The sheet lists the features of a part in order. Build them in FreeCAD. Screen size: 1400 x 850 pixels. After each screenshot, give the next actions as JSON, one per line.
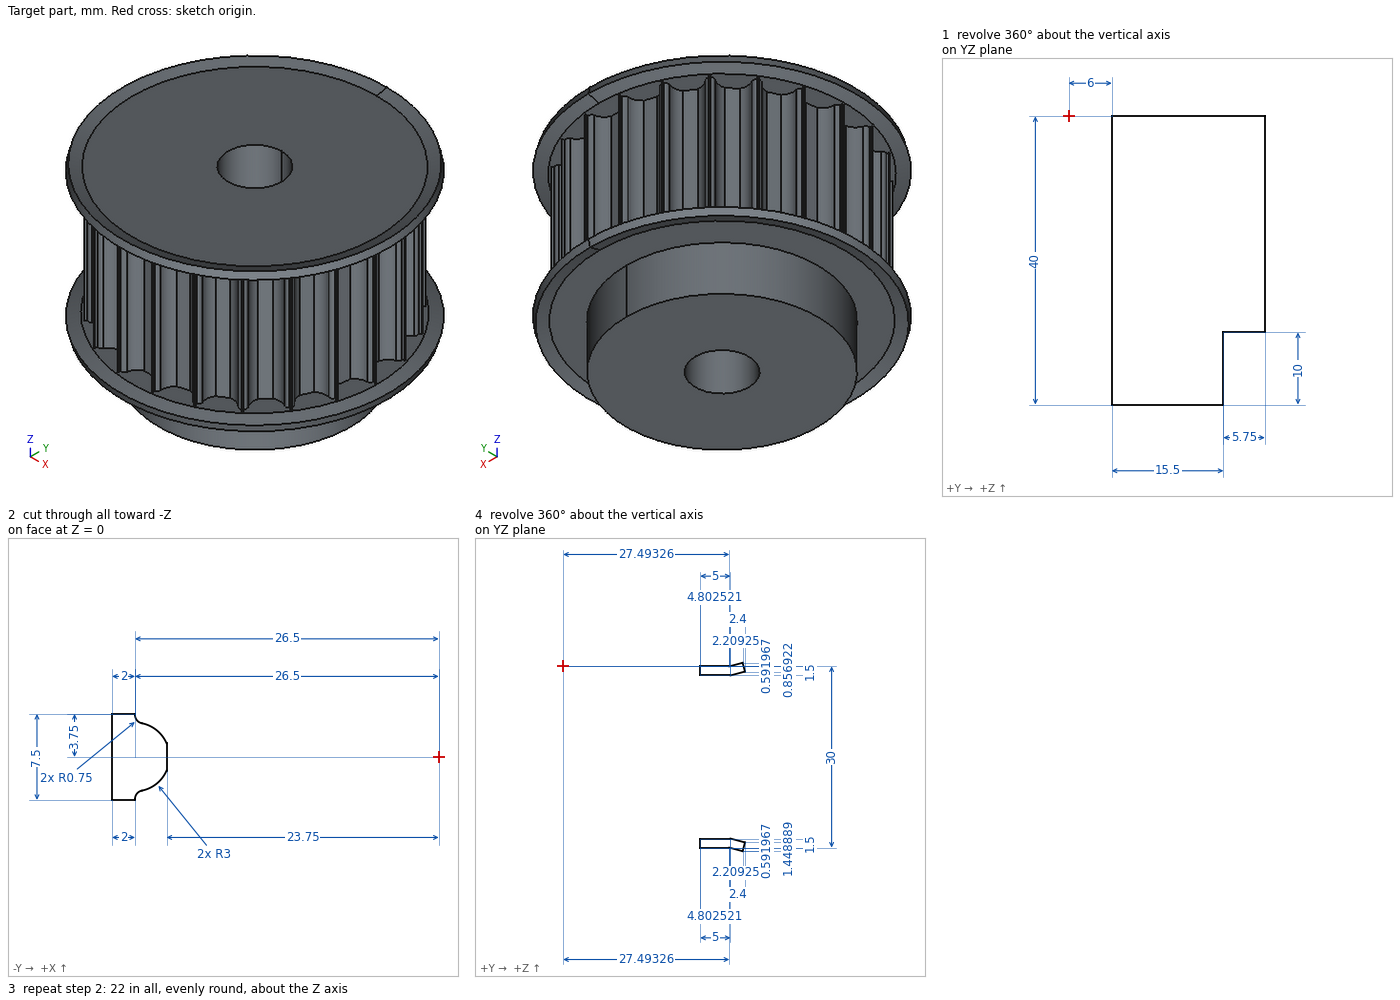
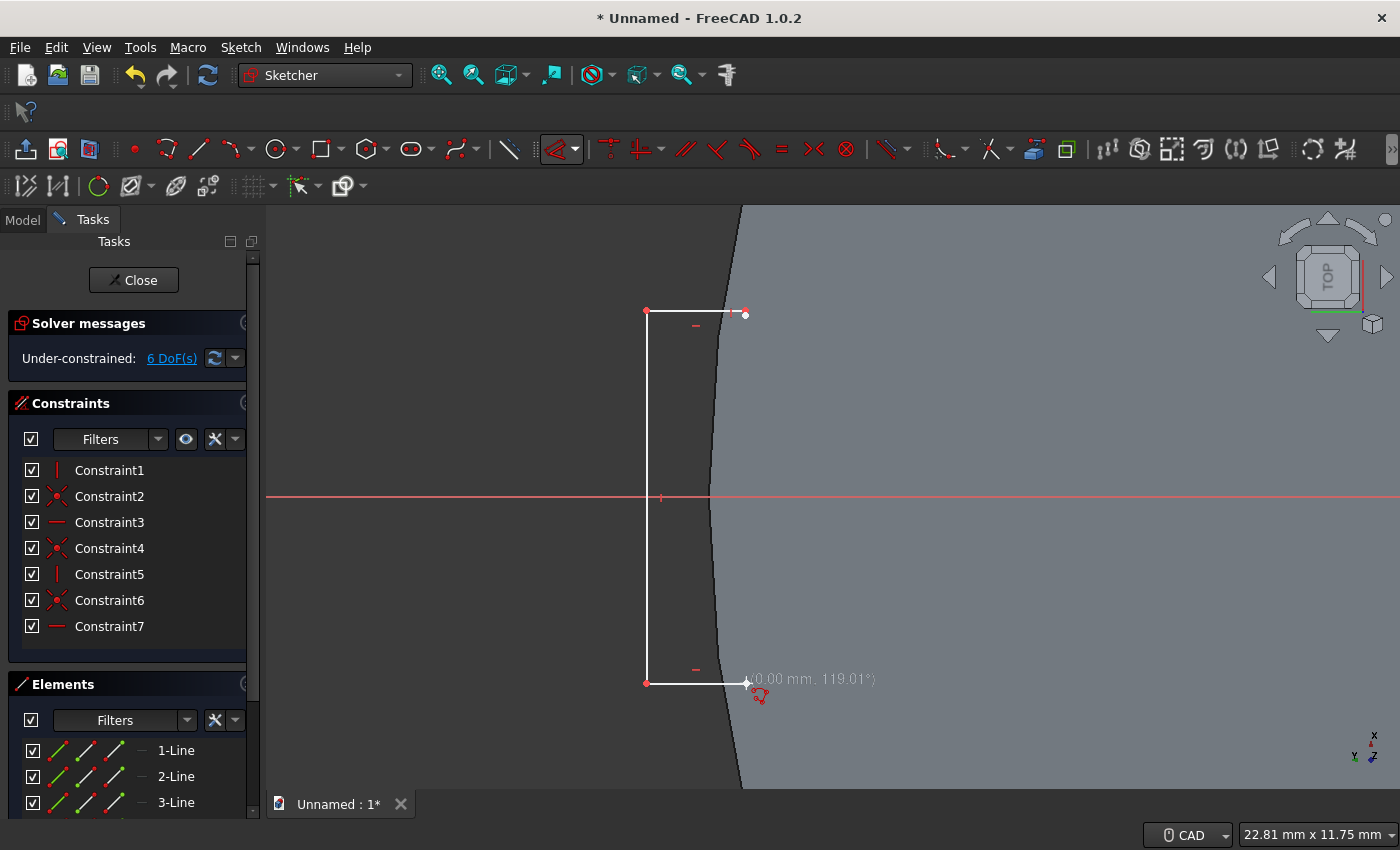
{"action": "scroll", "coordinate": [746, 680], "scroll_direction": "up", "scroll_amount": 8}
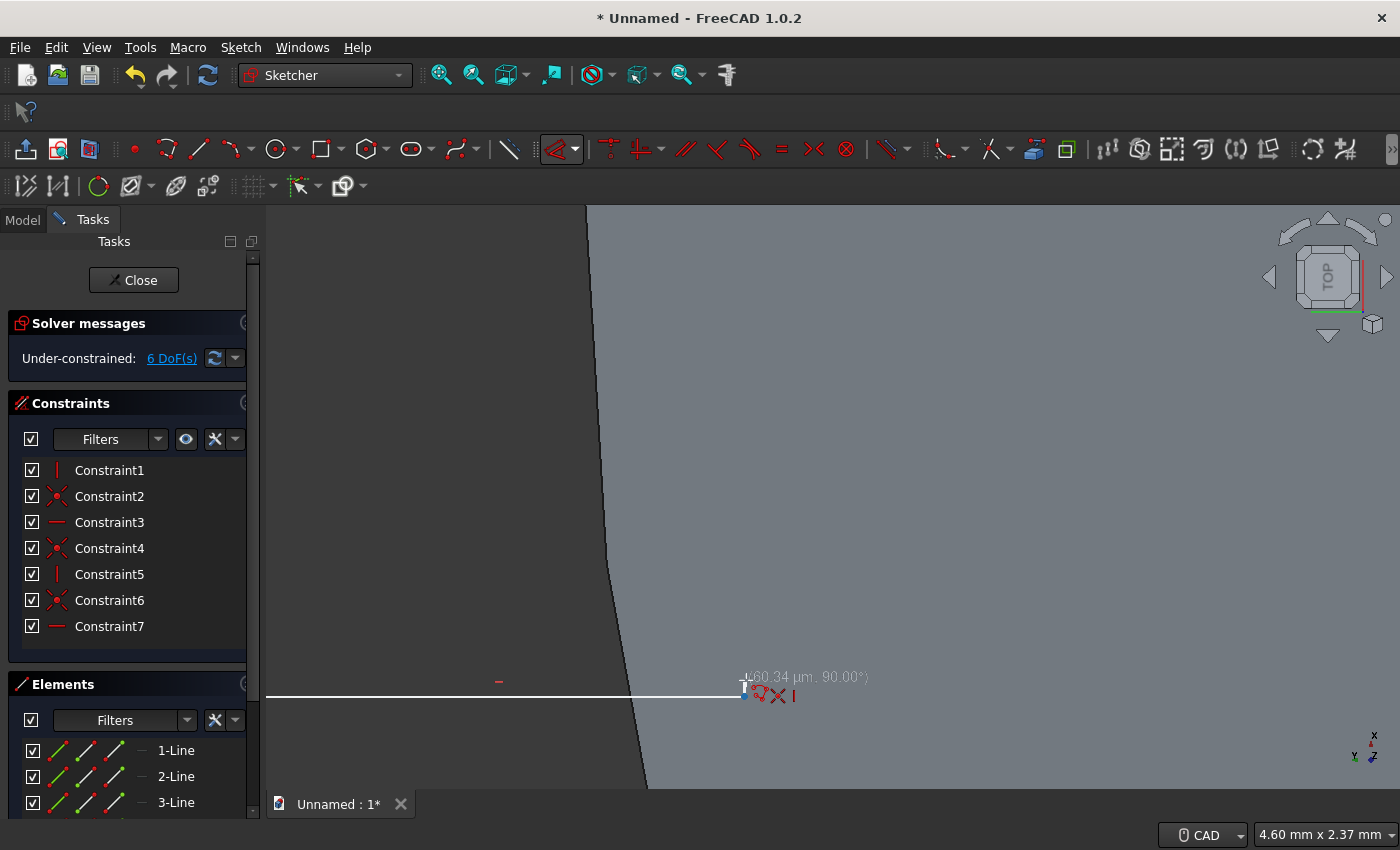
{"action": "left_click", "coordinate": [744, 675]}
{"action": "right_click", "coordinate": [744, 675]}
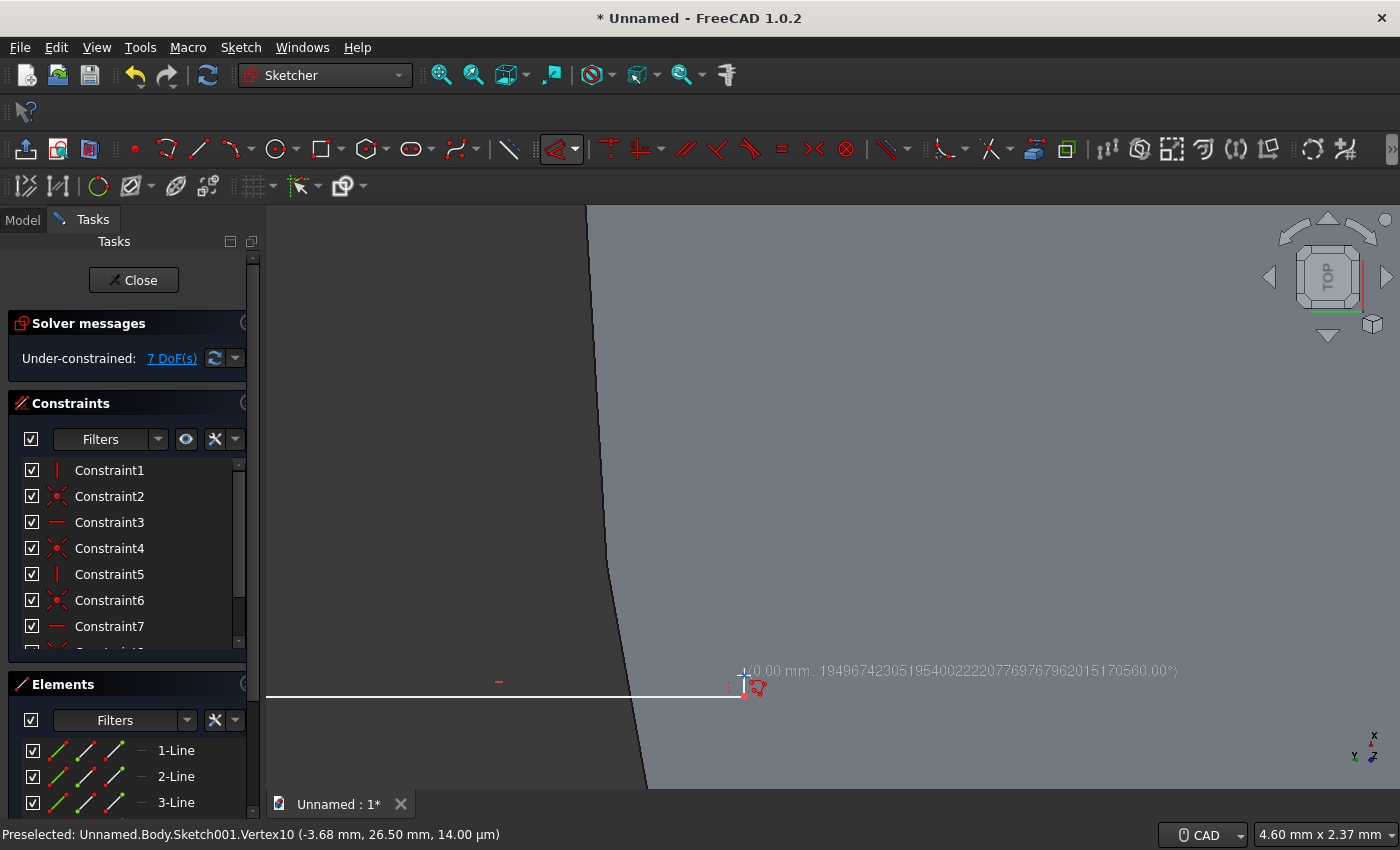
{"action": "key", "text": "g l"}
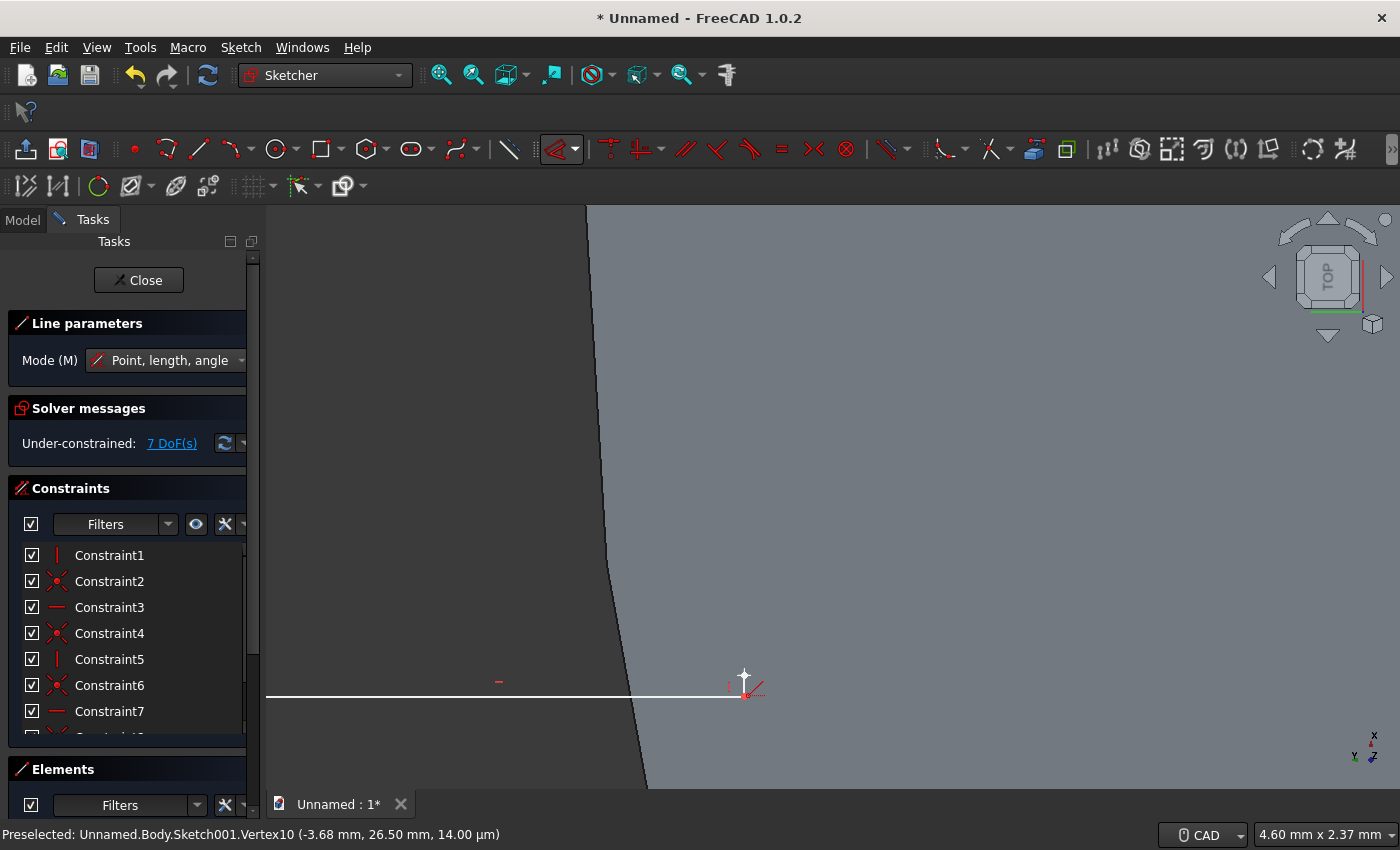
{"action": "scroll", "coordinate": [746, 681], "scroll_direction": "down", "scroll_amount": 8}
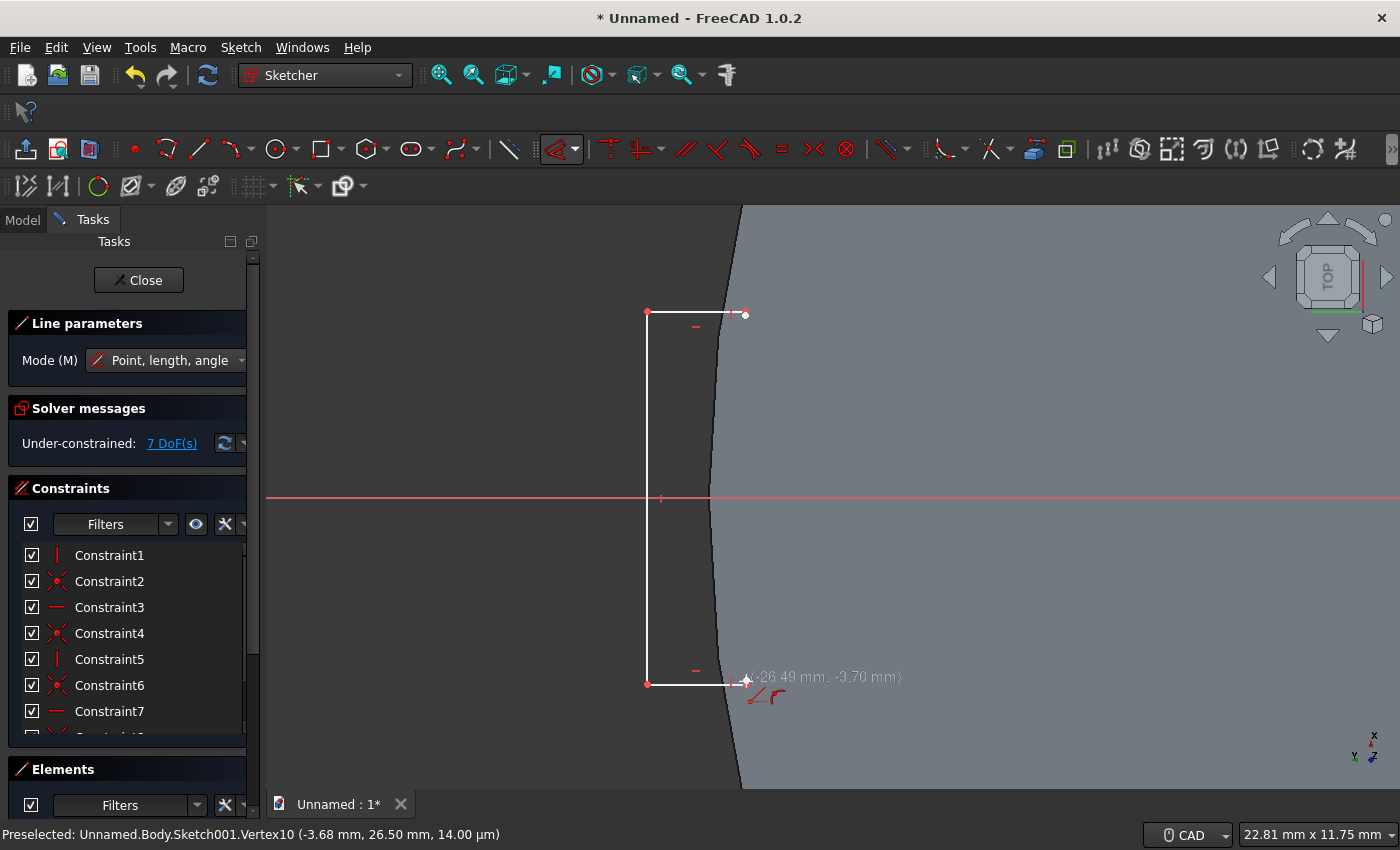
{"action": "left_click", "coordinate": [883, 557]}
{"action": "left_click", "coordinate": [883, 438]}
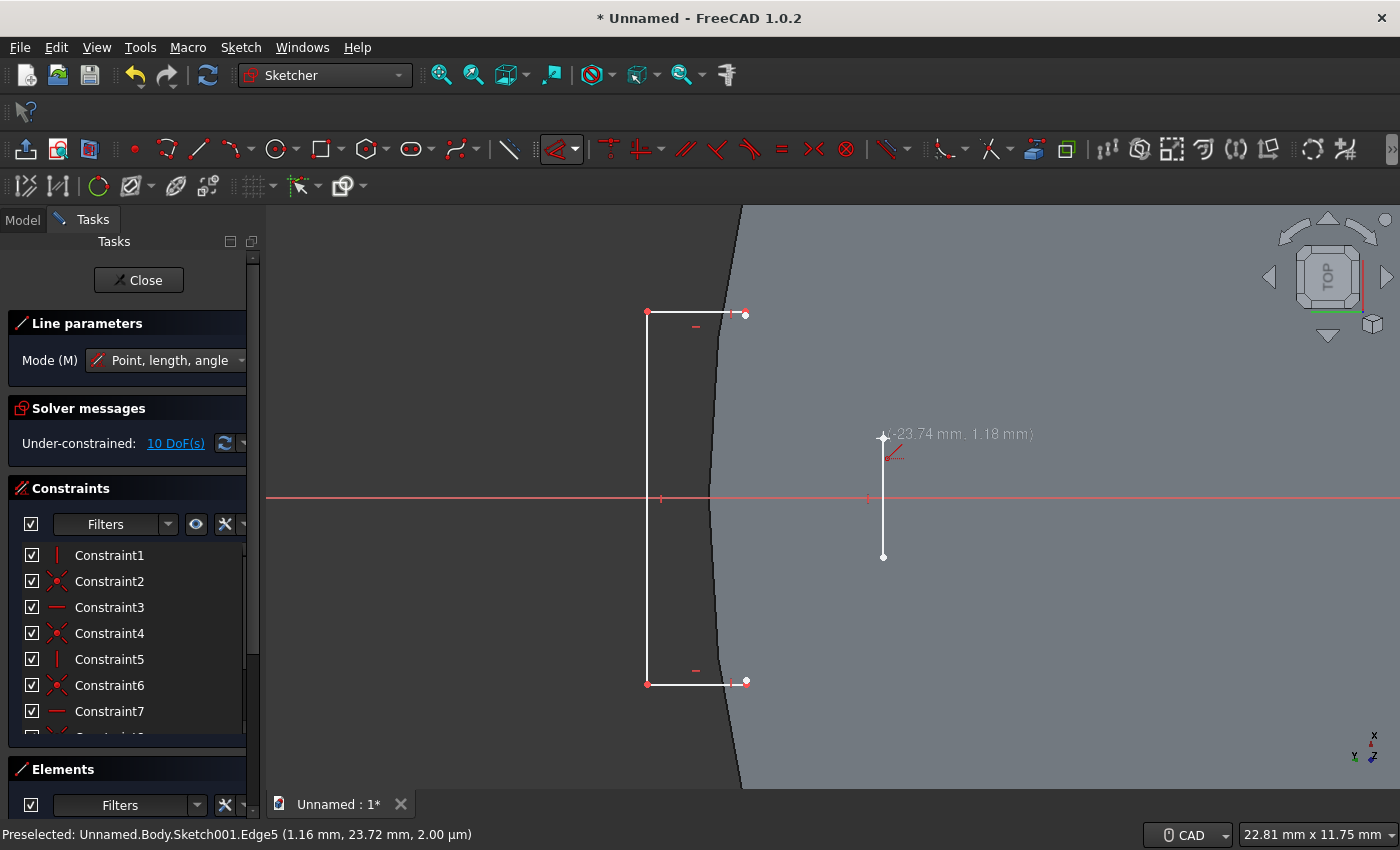
{"action": "left_click", "coordinate": [232, 150]}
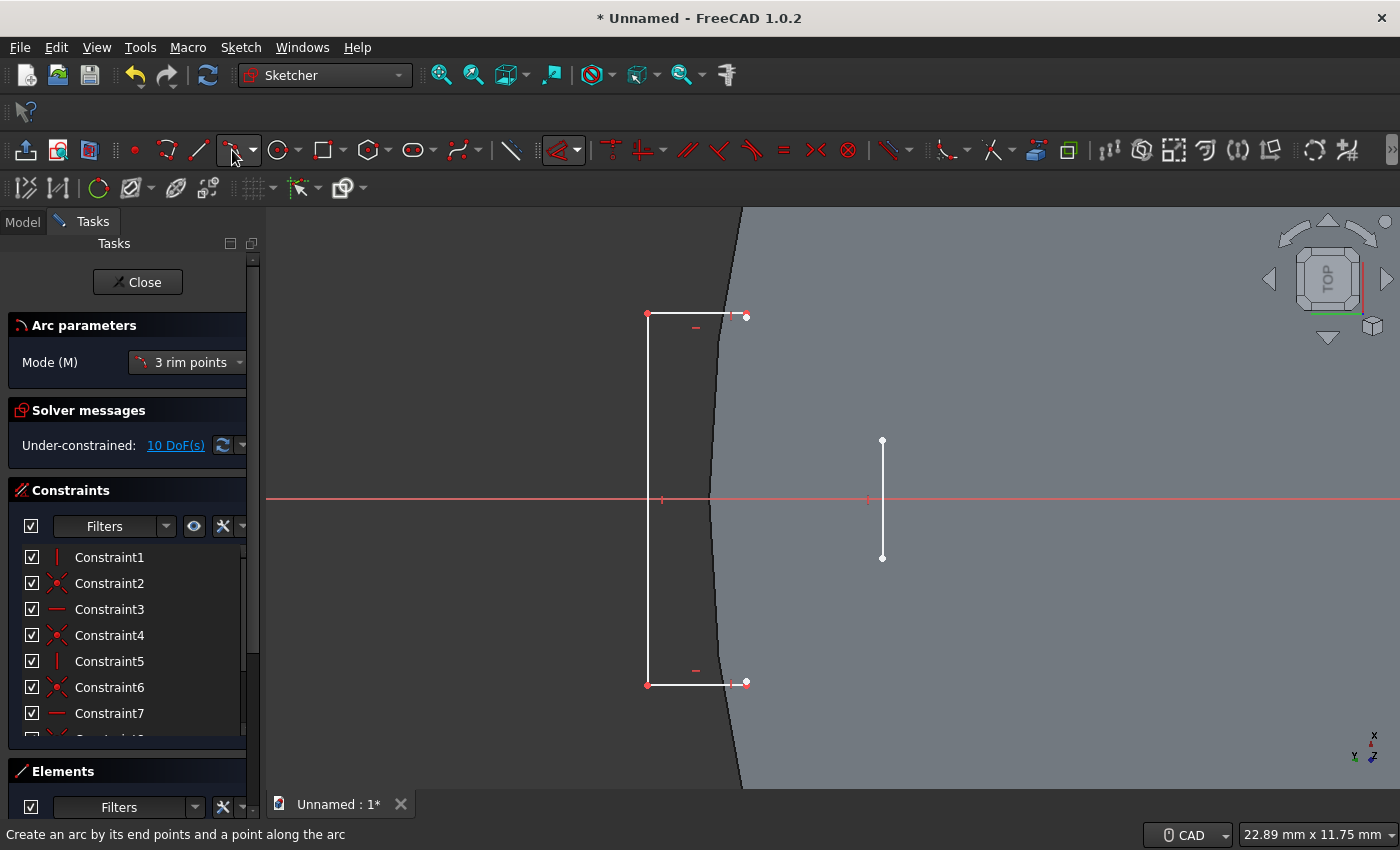
{"action": "scroll", "coordinate": [746, 681], "scroll_direction": "up", "scroll_amount": 11}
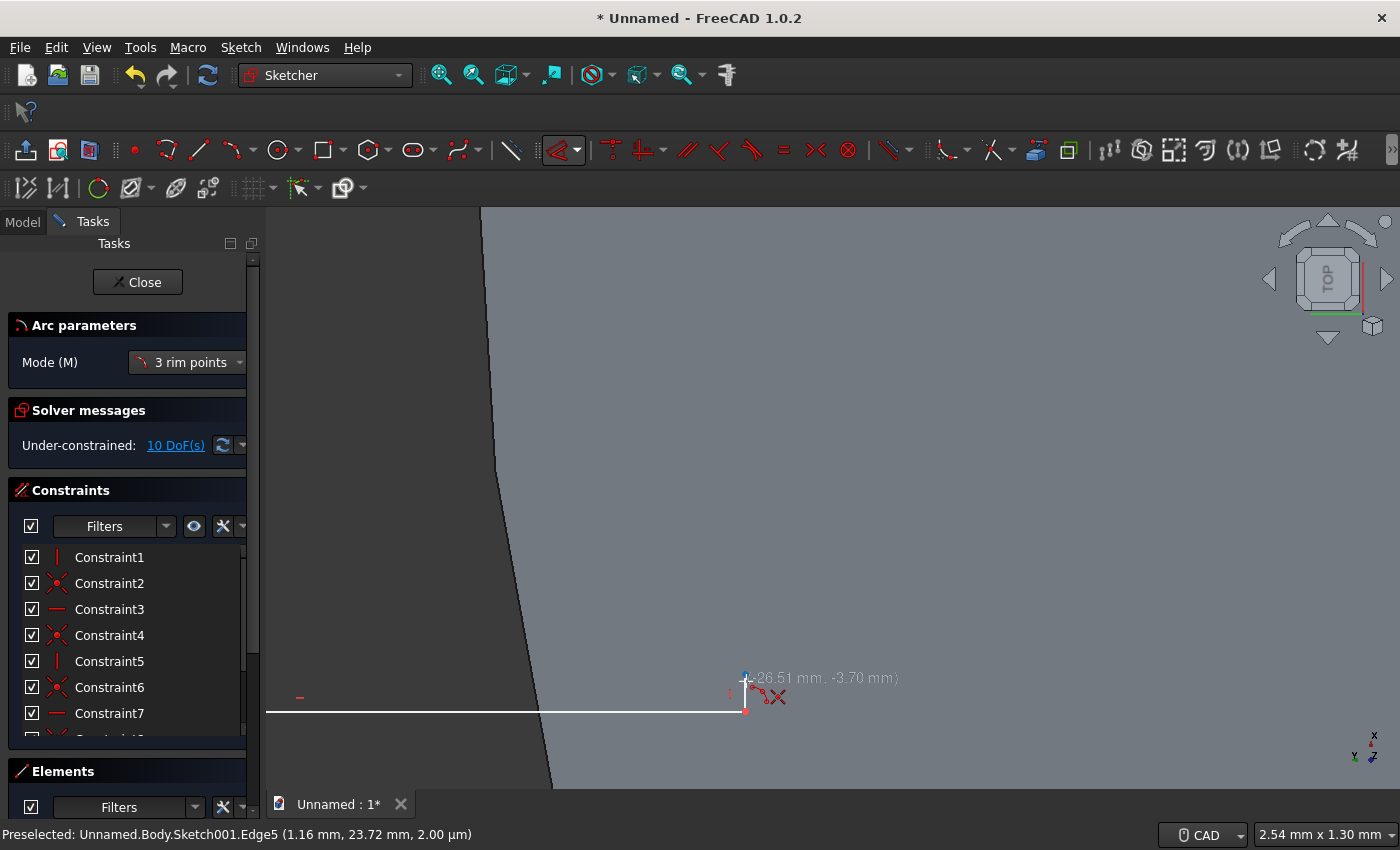
{"action": "left_click", "coordinate": [745, 675]}